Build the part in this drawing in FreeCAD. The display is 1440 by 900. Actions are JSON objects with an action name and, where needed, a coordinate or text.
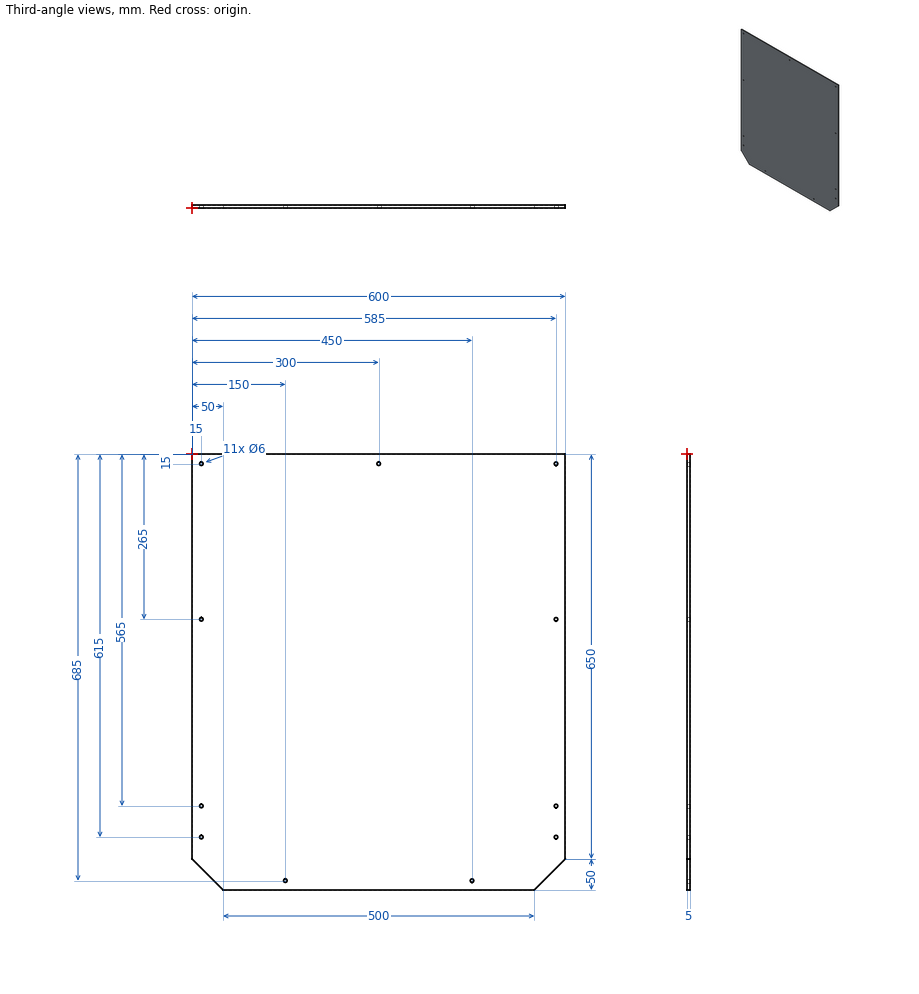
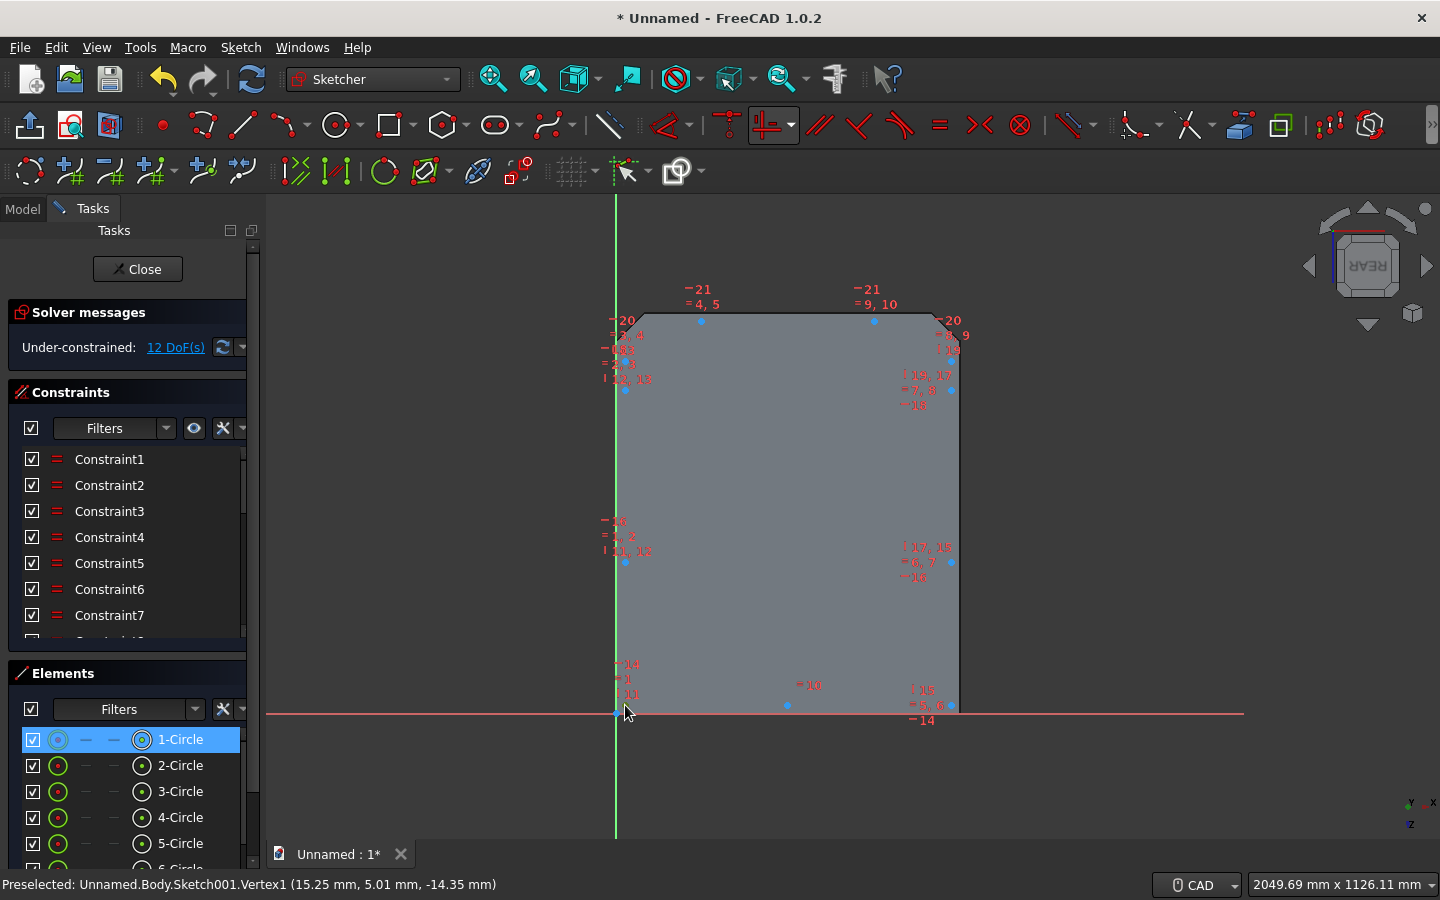
{"action": "left_click", "coordinate": [788, 705]}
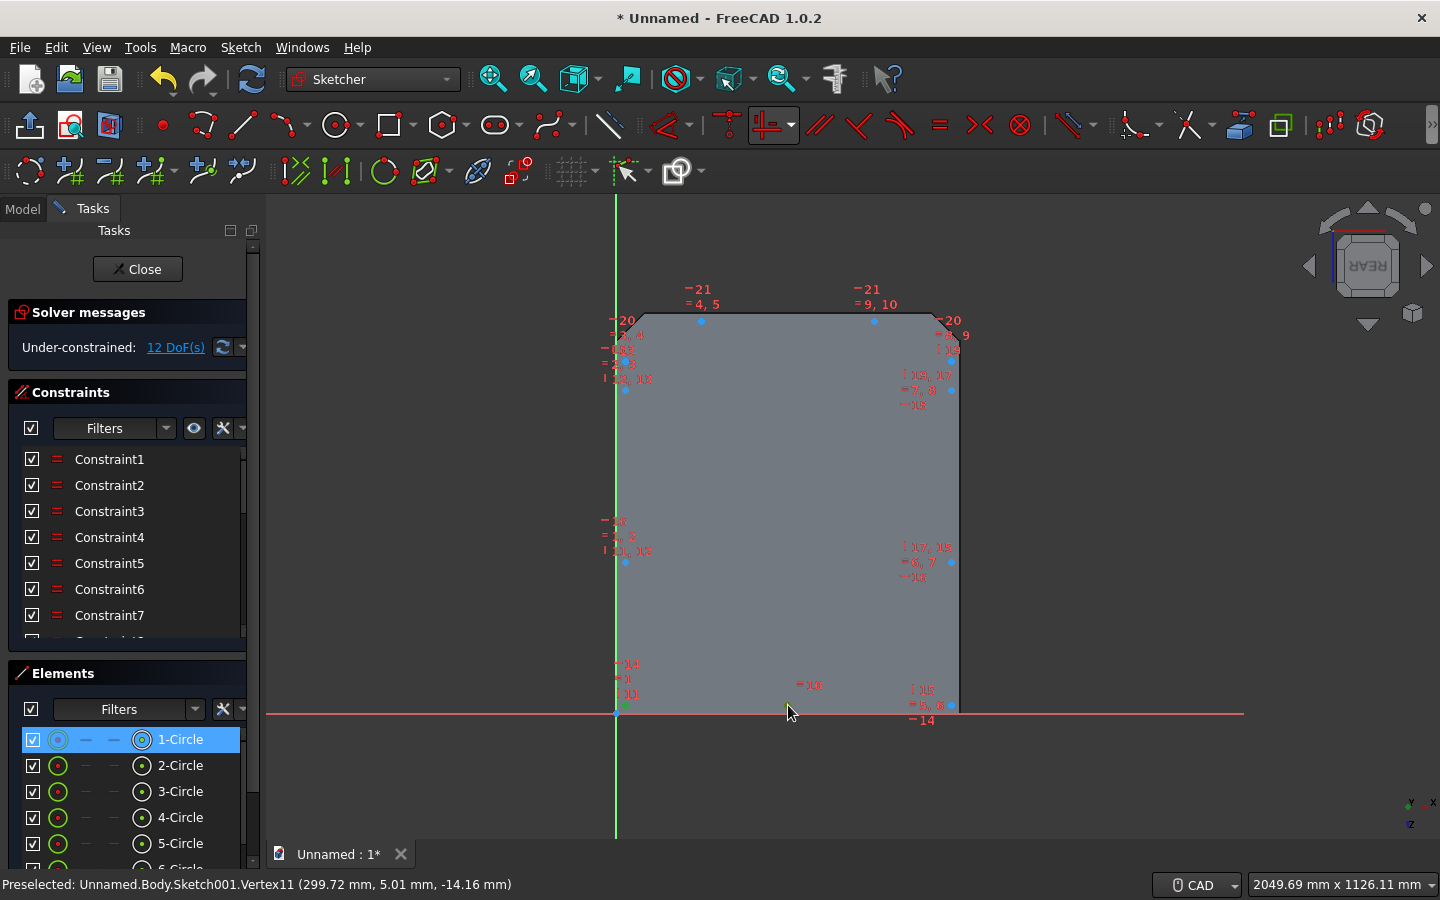
{"action": "key", "text": "h"}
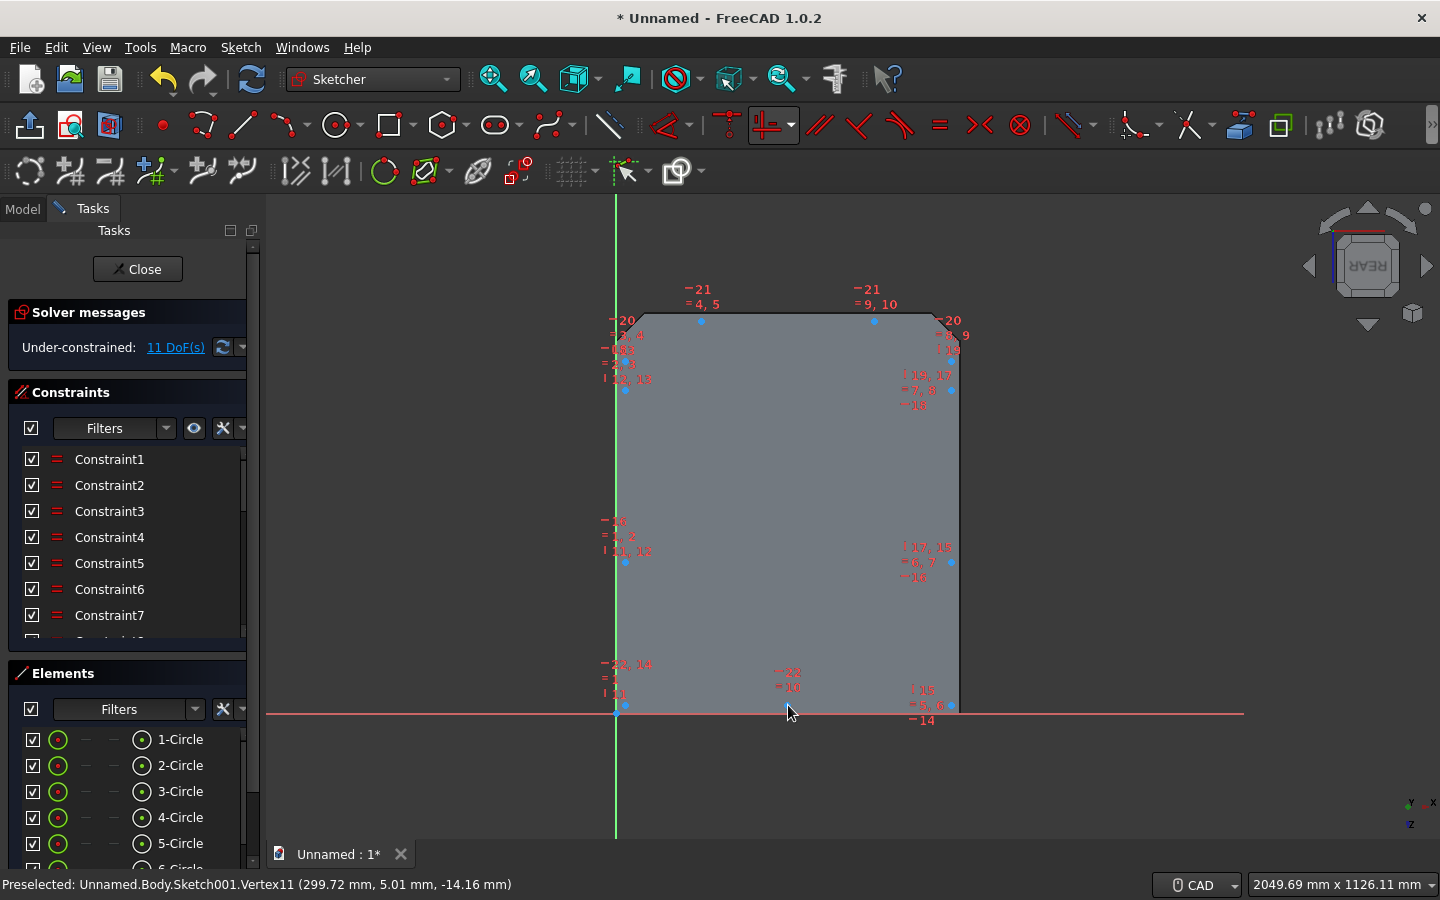
{"action": "left_click", "coordinate": [664, 126]}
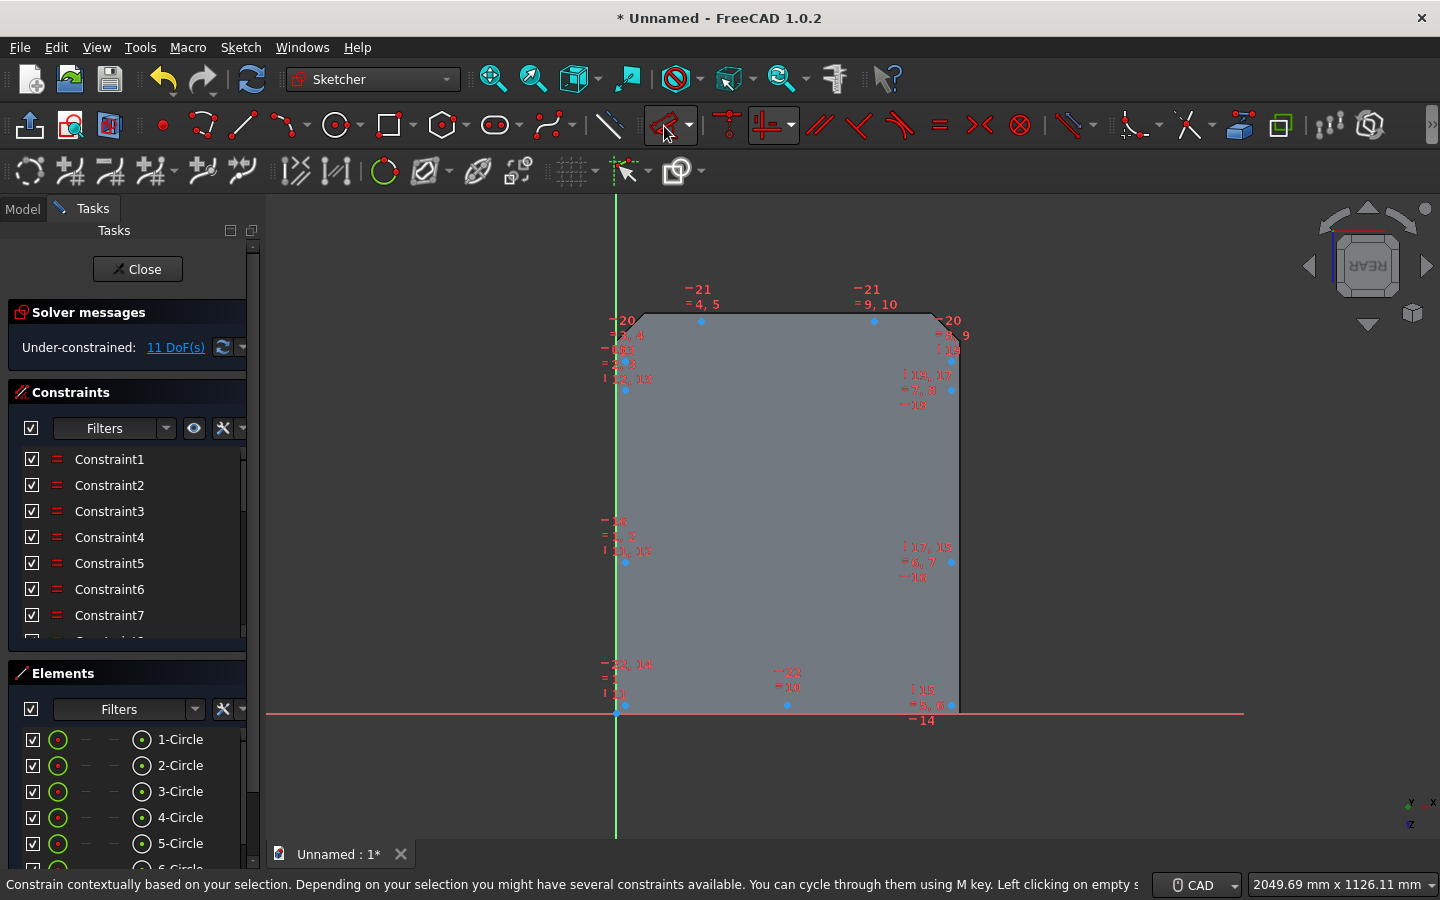
{"action": "scroll", "coordinate": [626, 704], "scroll_direction": "up", "scroll_amount": 13}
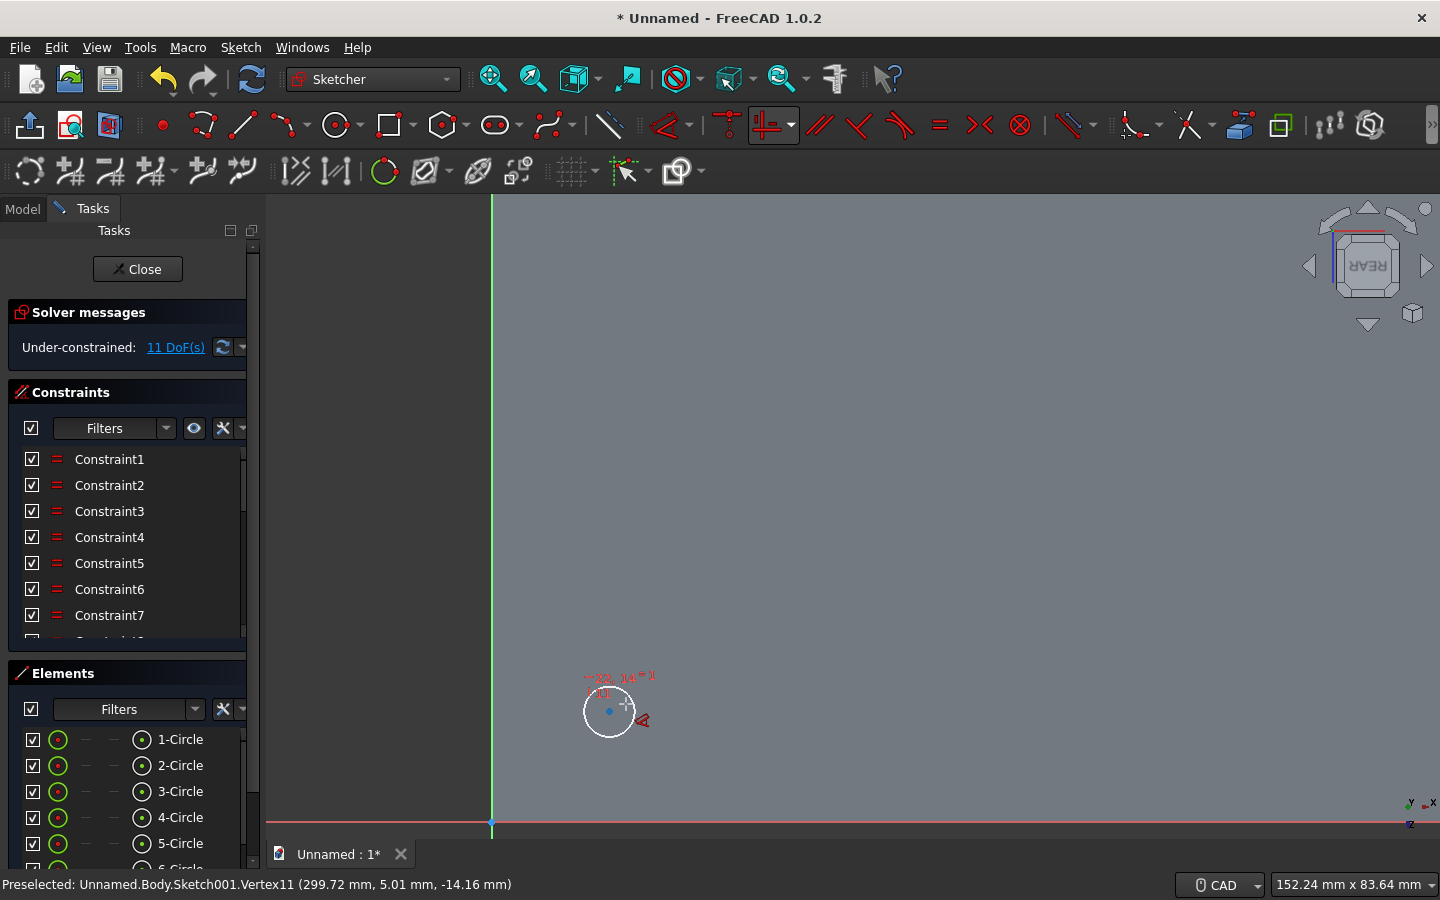
{"action": "left_click", "coordinate": [627, 694]}
{"action": "left_click", "coordinate": [650, 671]}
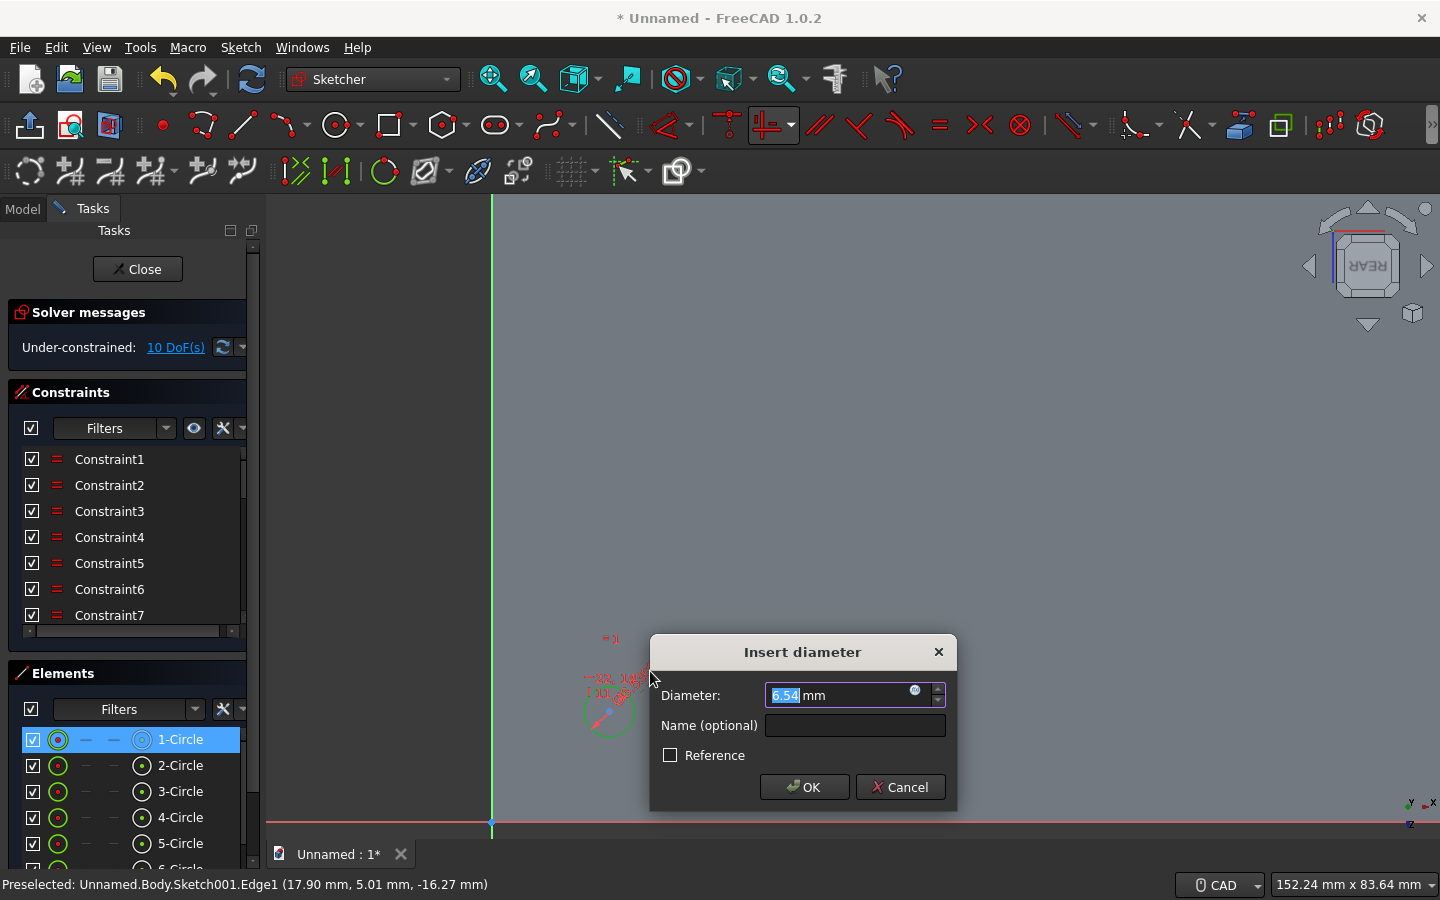
{"action": "type", "text": "6"}
{"action": "key", "text": "Return"}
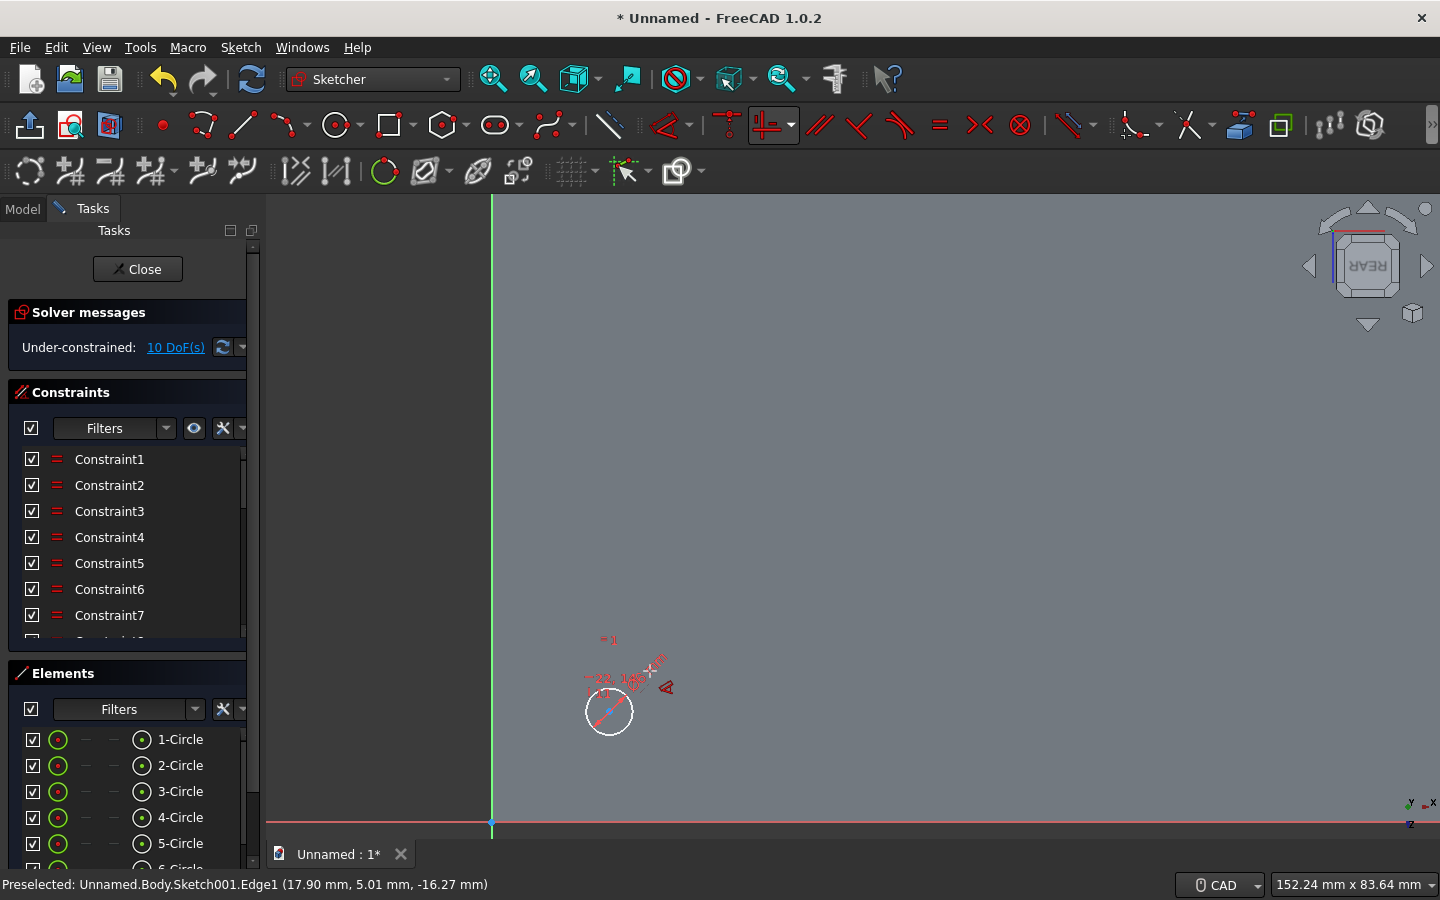
{"action": "scroll", "coordinate": [626, 705], "scroll_direction": "down", "scroll_amount": 13}